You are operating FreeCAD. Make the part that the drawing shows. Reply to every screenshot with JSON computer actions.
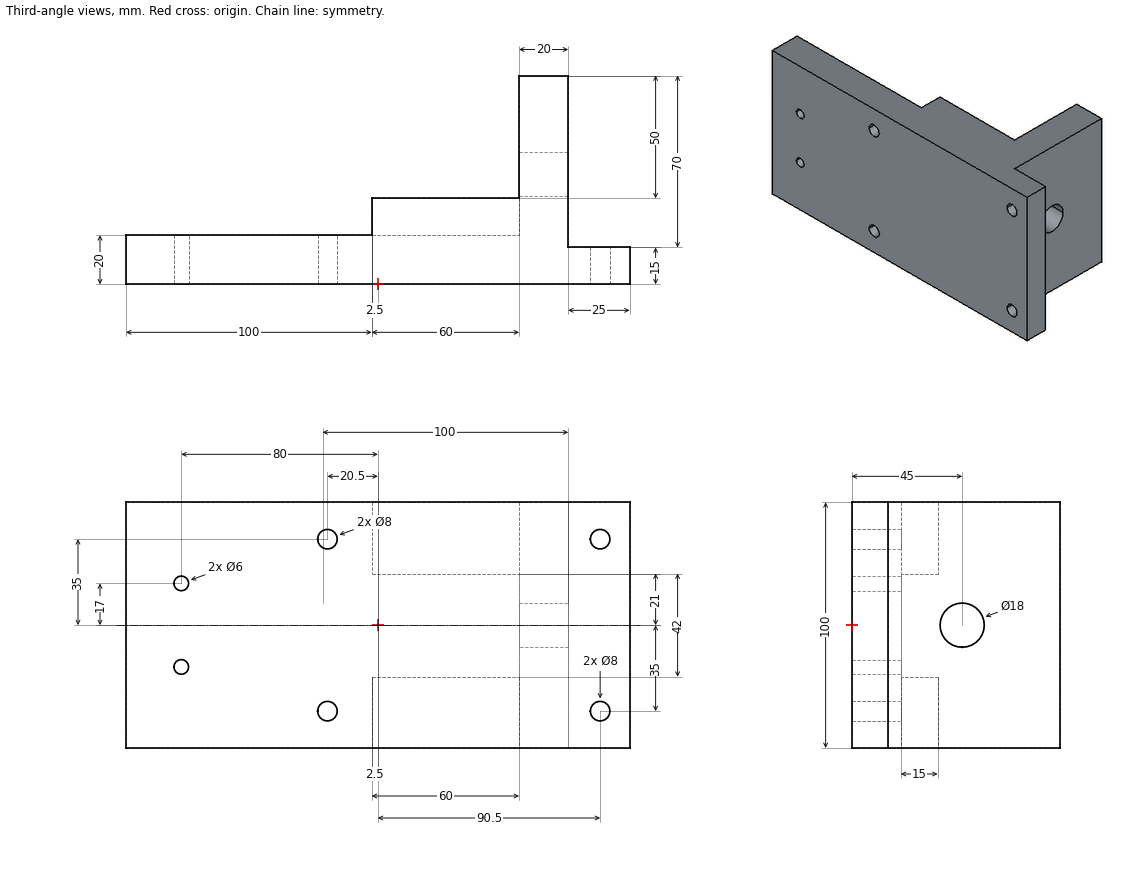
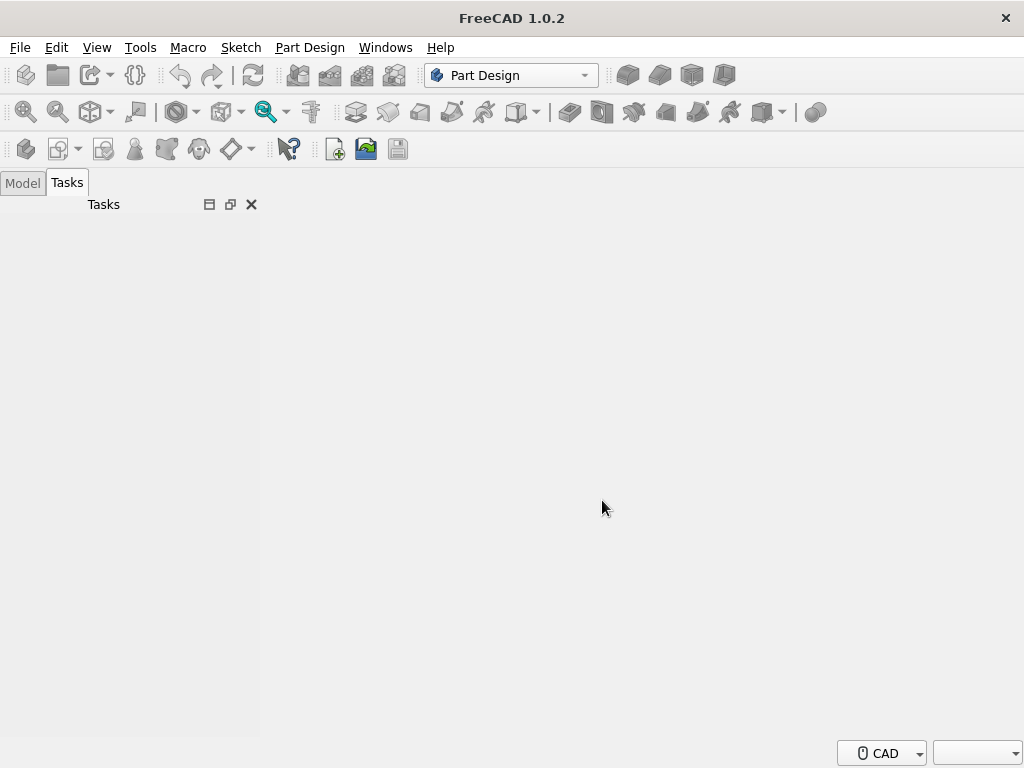
{"action": "left_click", "coordinate": [334, 150]}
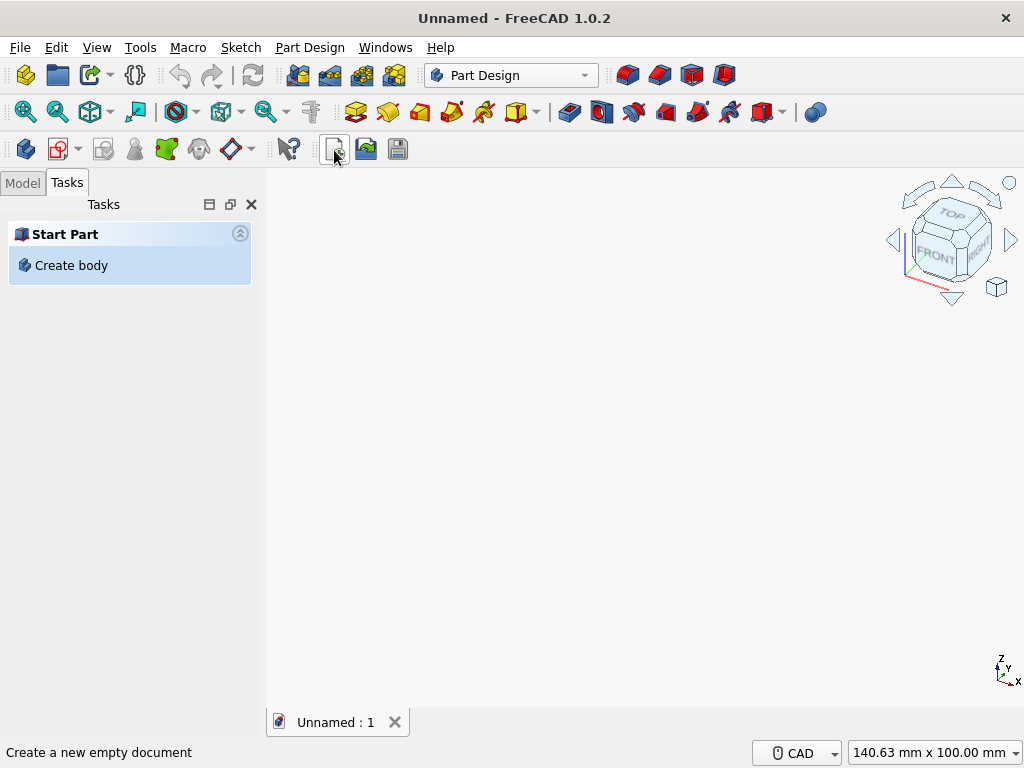
{"action": "left_click", "coordinate": [58, 150]}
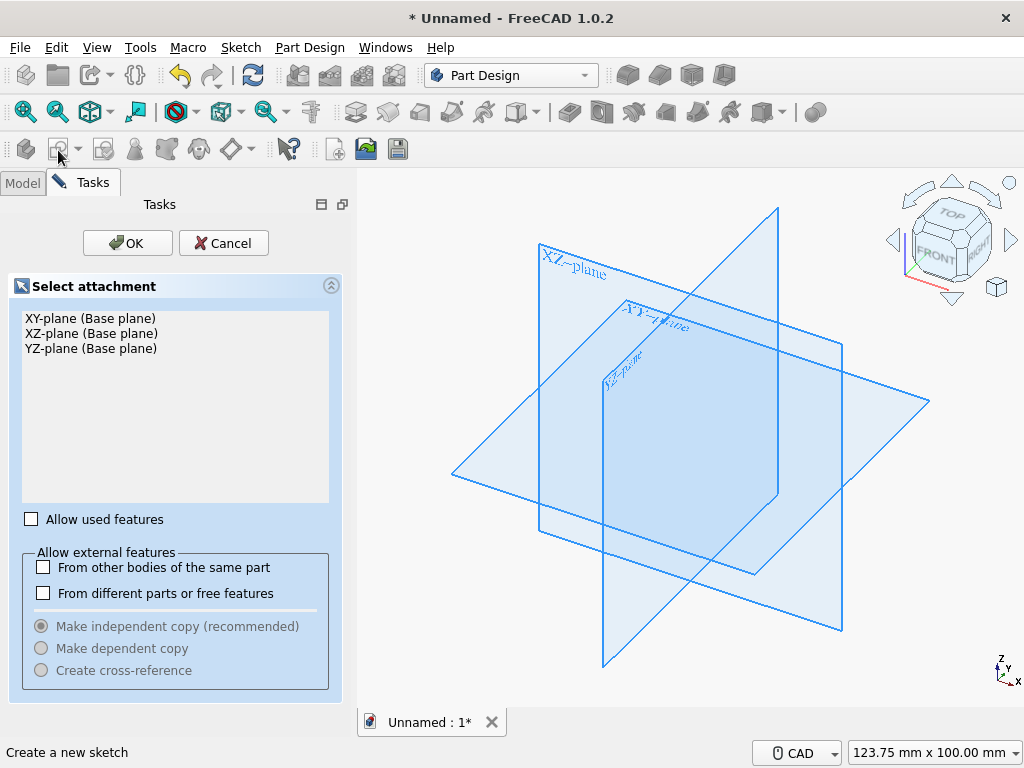
{"action": "left_click", "coordinate": [82, 318]}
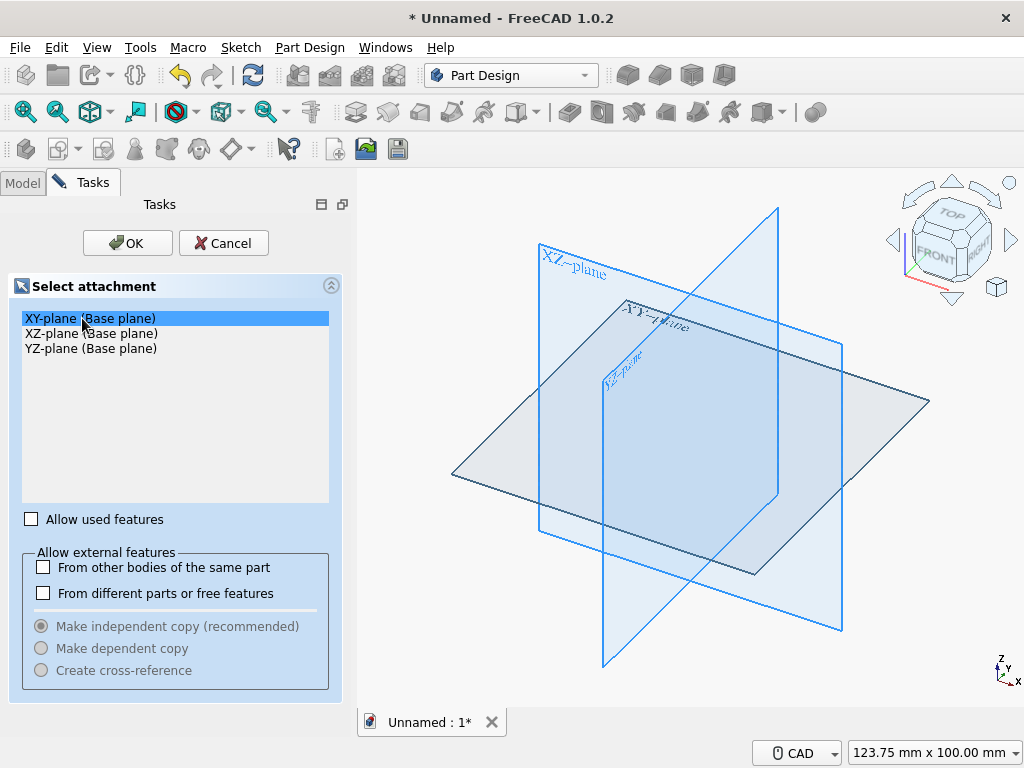
{"action": "left_click", "coordinate": [128, 243]}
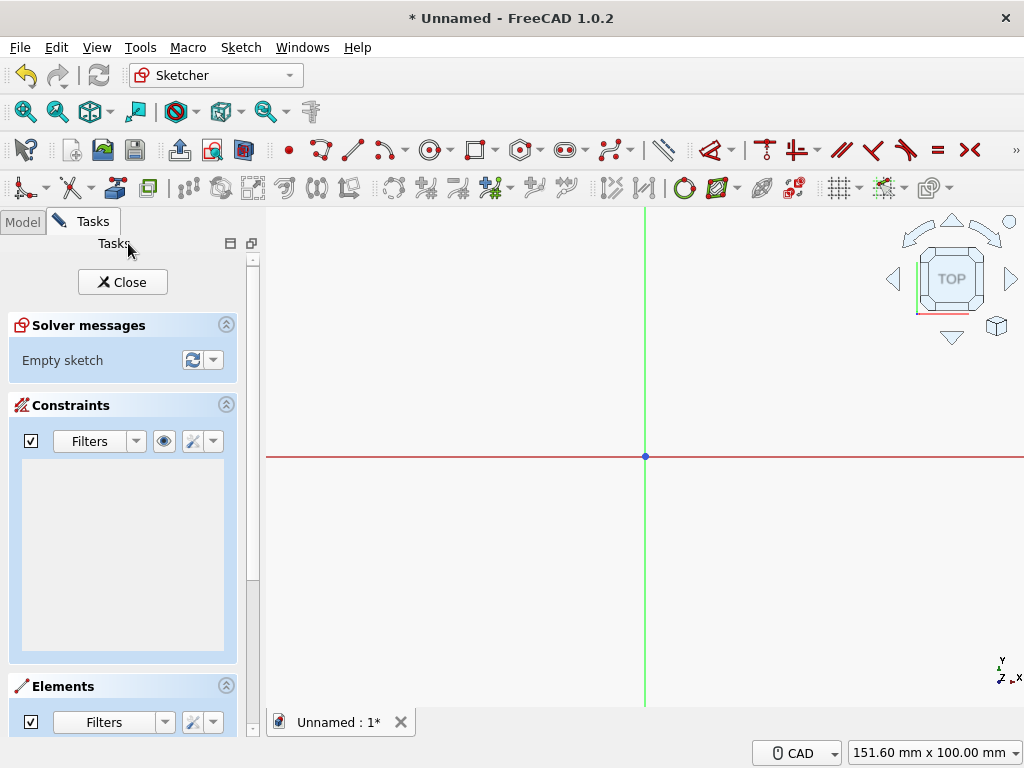
{"action": "scroll", "coordinate": [537, 581], "scroll_direction": "down", "scroll_amount": 5}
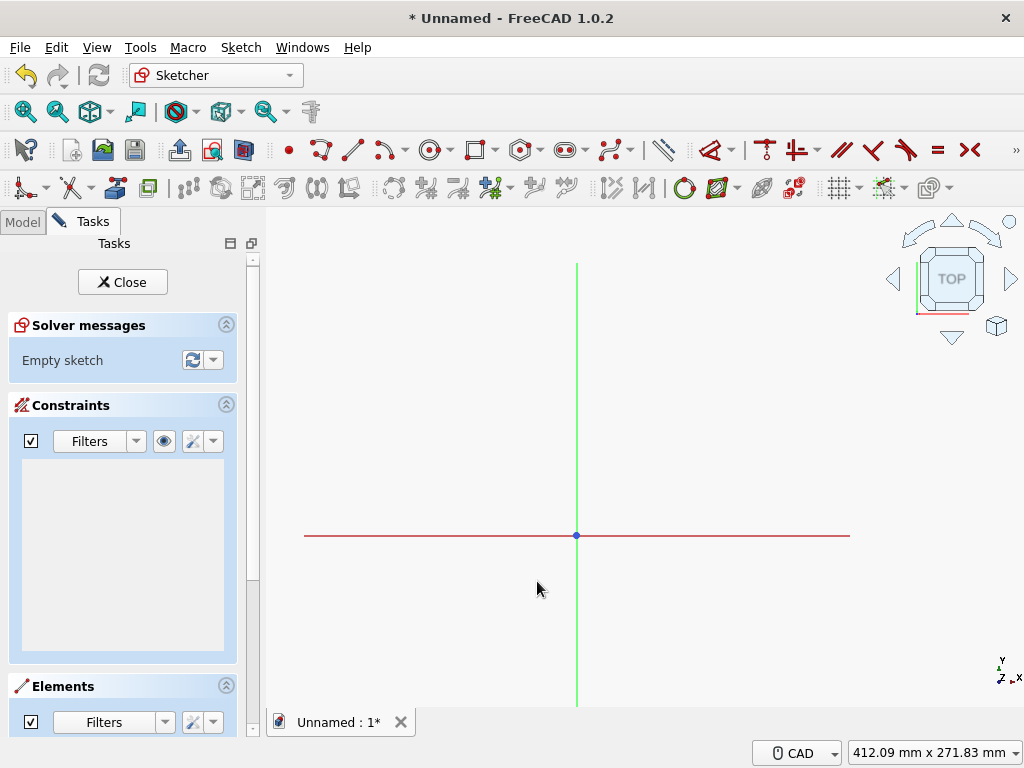
{"action": "left_click", "coordinate": [322, 150]}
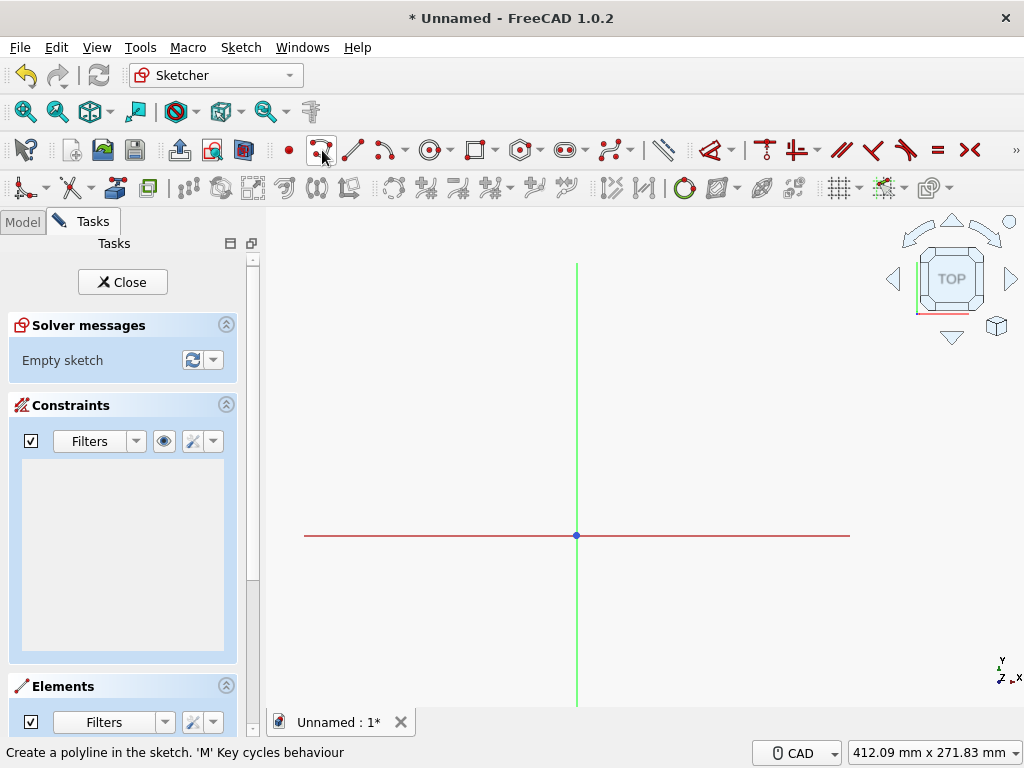
{"action": "scroll", "coordinate": [572, 499], "scroll_direction": "up", "scroll_amount": 7}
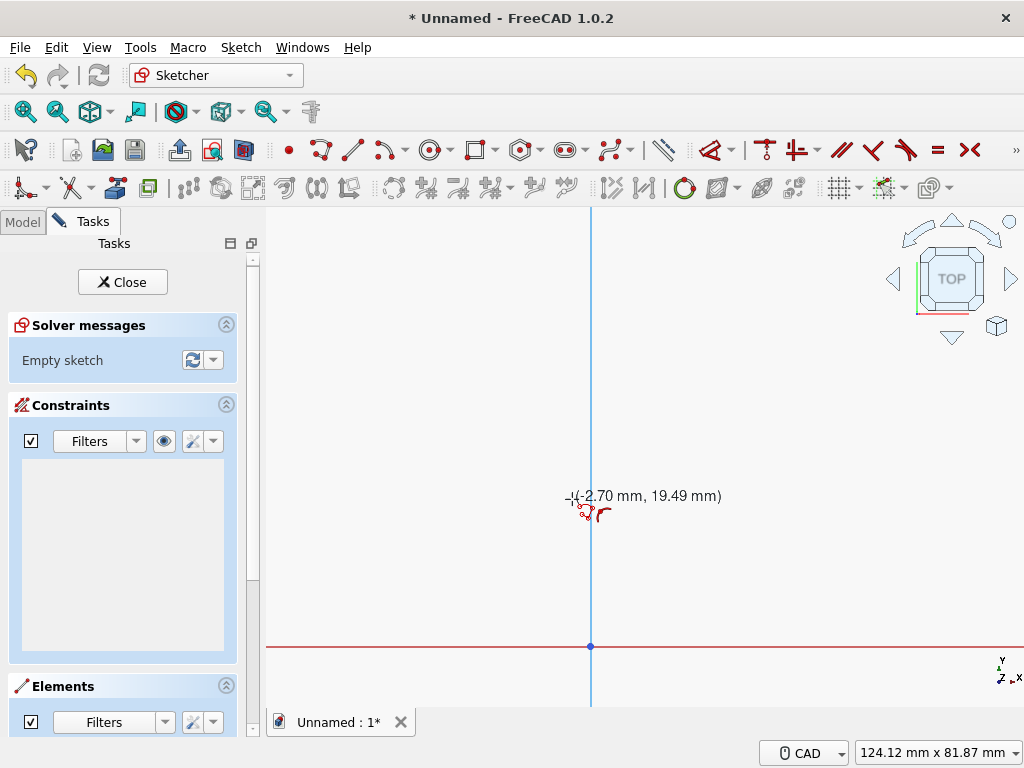
{"action": "left_click", "coordinate": [572, 497]}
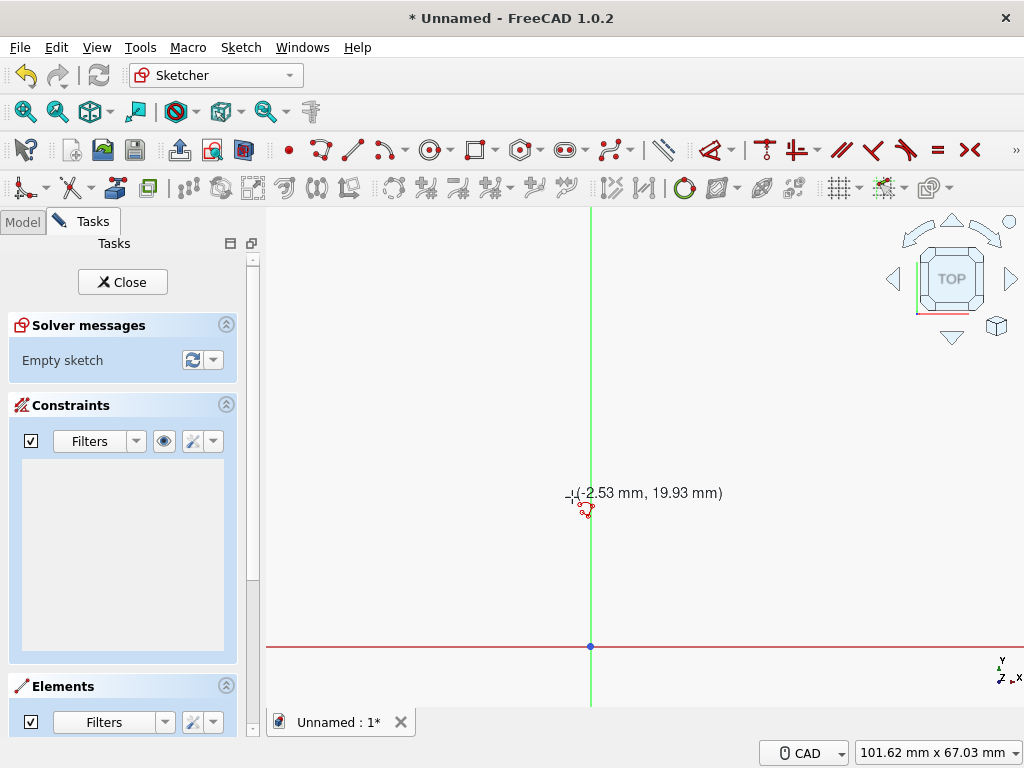
{"action": "scroll", "coordinate": [572, 499], "scroll_direction": "down", "scroll_amount": 7}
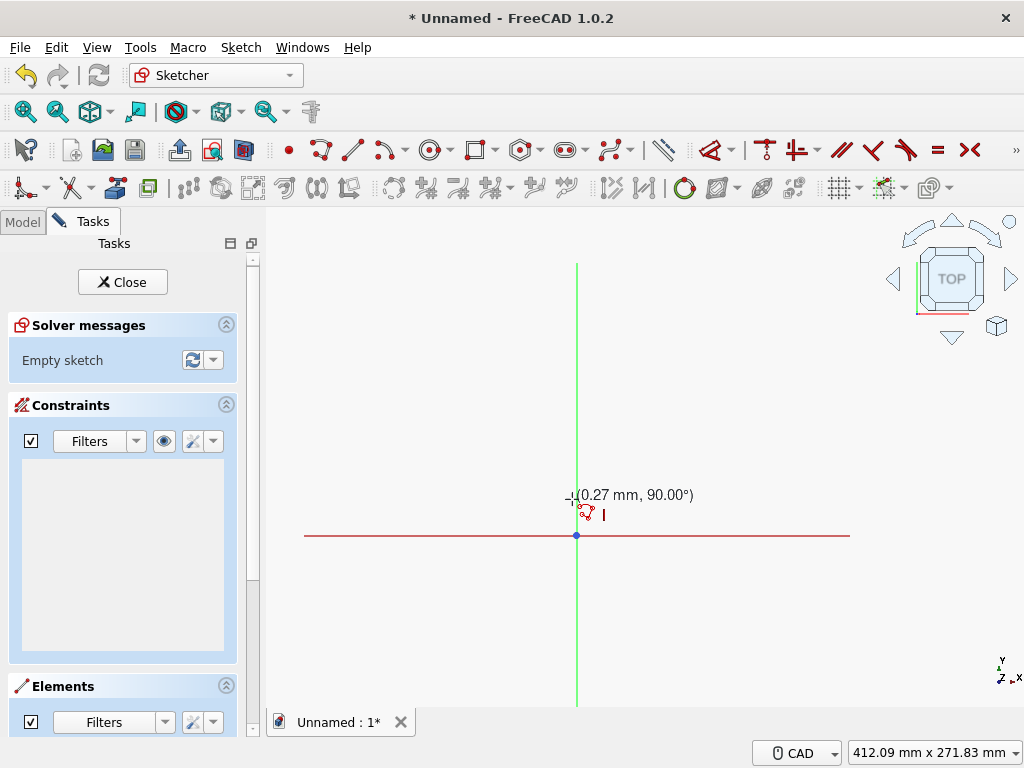
{"action": "left_click", "coordinate": [388, 499]}
{"action": "left_click", "coordinate": [388, 536]}
{"action": "left_click", "coordinate": [765, 527]}
{"action": "left_click", "coordinate": [765, 508]}
{"action": "left_click", "coordinate": [720, 508]}
{"action": "left_click", "coordinate": [720, 380]}
{"action": "left_click", "coordinate": [683, 380]}
{"action": "left_click", "coordinate": [683, 471]}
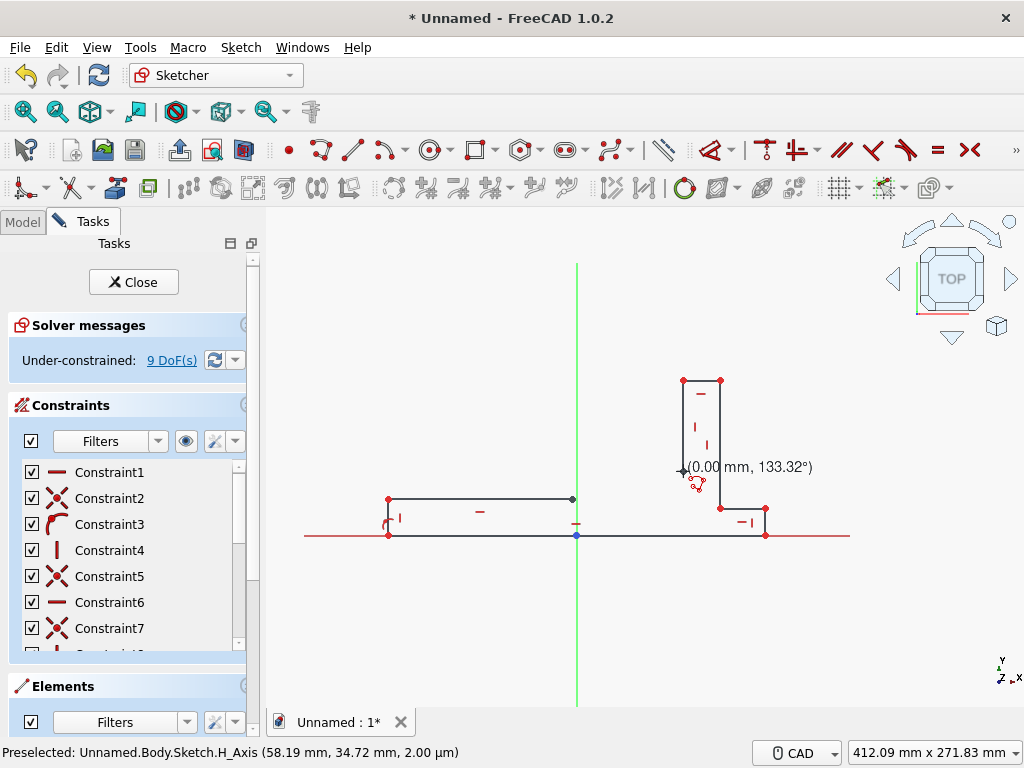
{"action": "scroll", "coordinate": [572, 471], "scroll_direction": "up", "scroll_amount": 7}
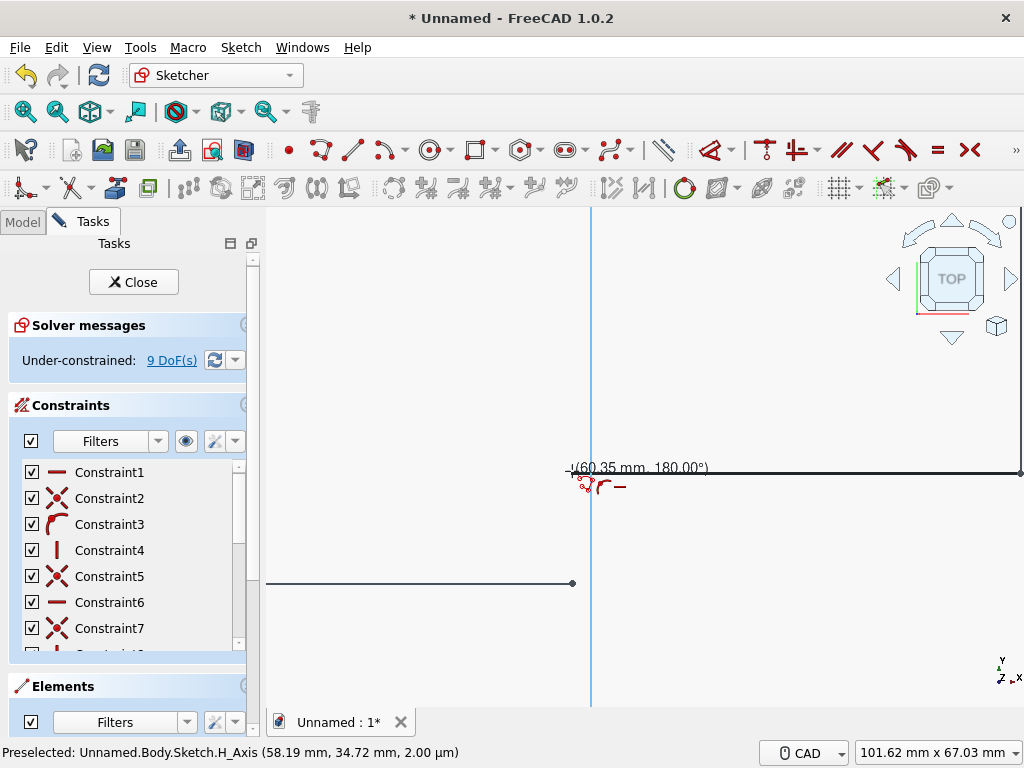
{"action": "left_click", "coordinate": [572, 469]}
{"action": "left_click", "coordinate": [572, 584]}
{"action": "key", "text": "Escape"}
{"action": "key", "text": "Escape"}